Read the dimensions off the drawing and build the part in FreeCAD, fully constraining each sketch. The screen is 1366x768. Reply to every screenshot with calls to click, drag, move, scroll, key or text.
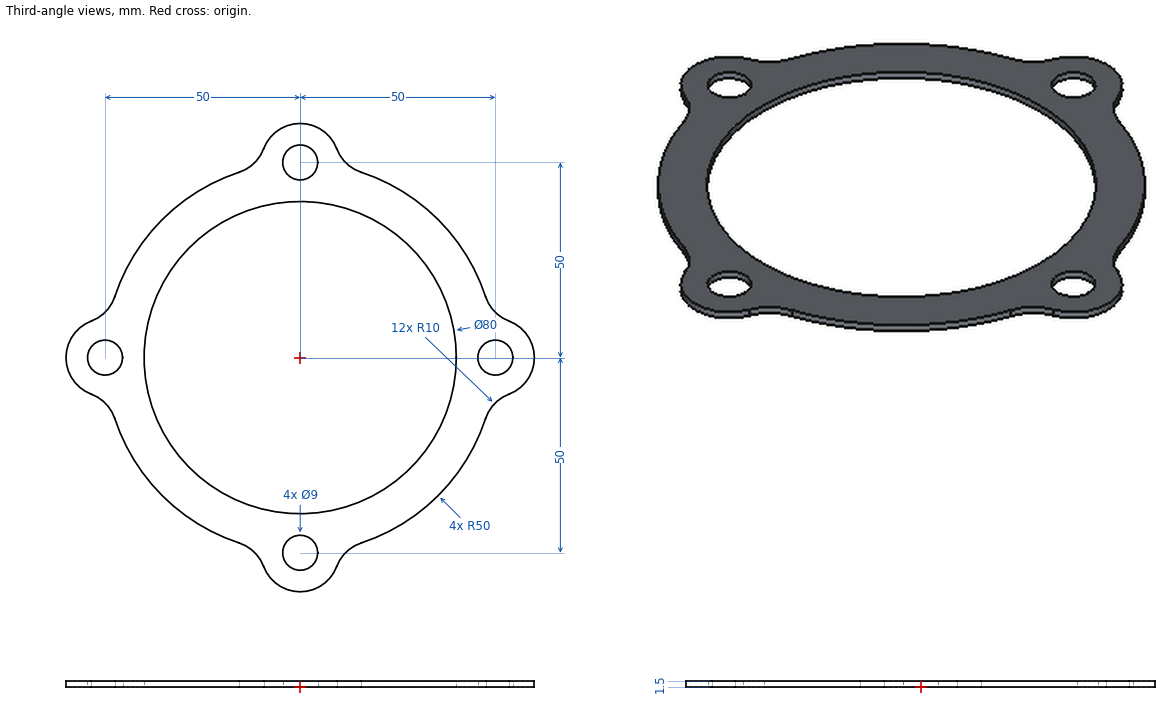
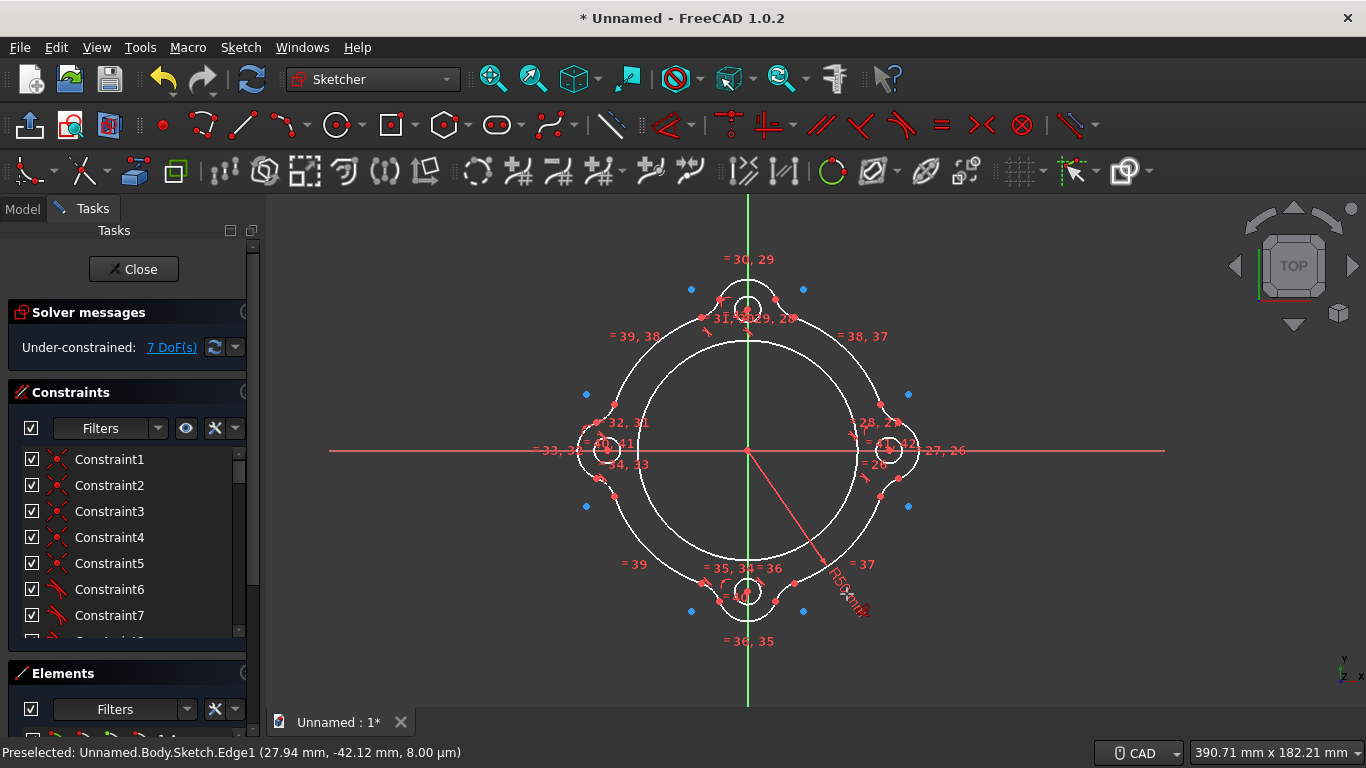
scroll(888, 486, up, 2)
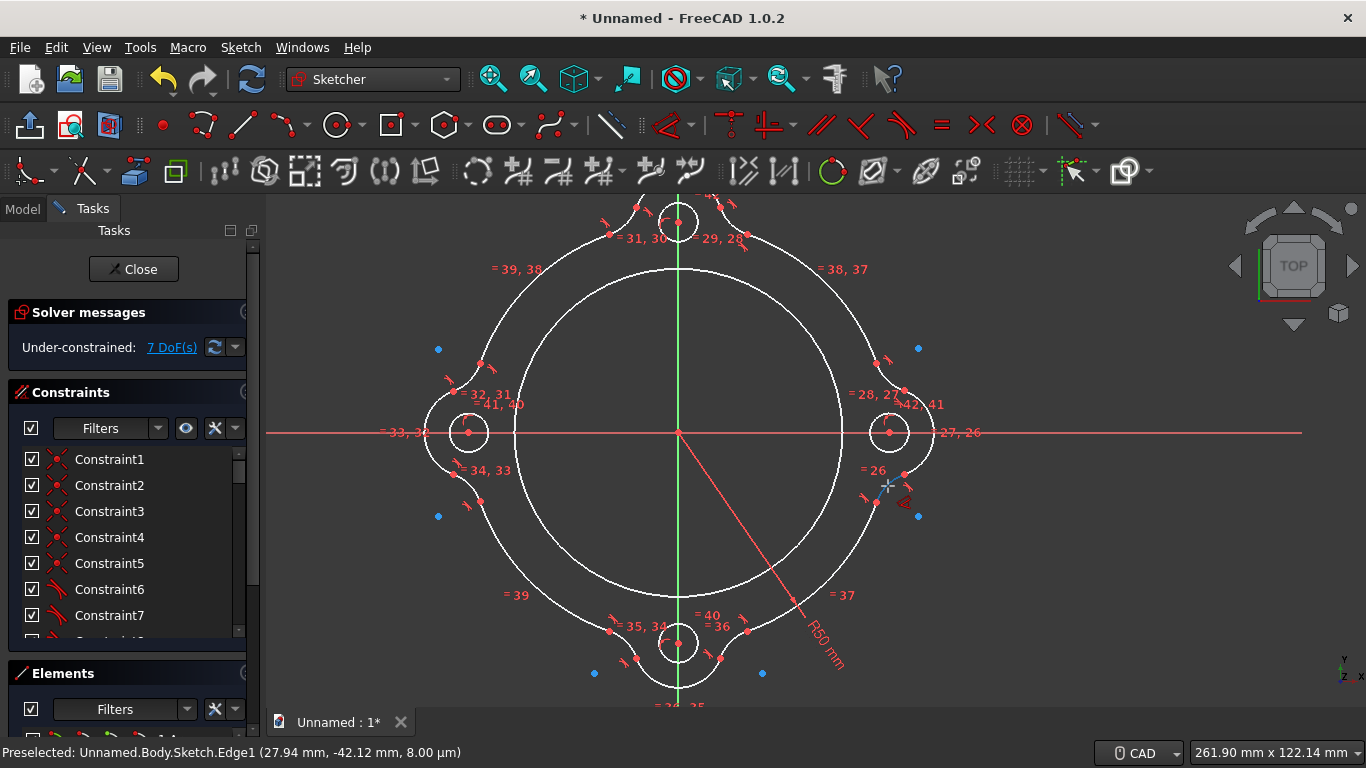
click(887, 485)
click(864, 462)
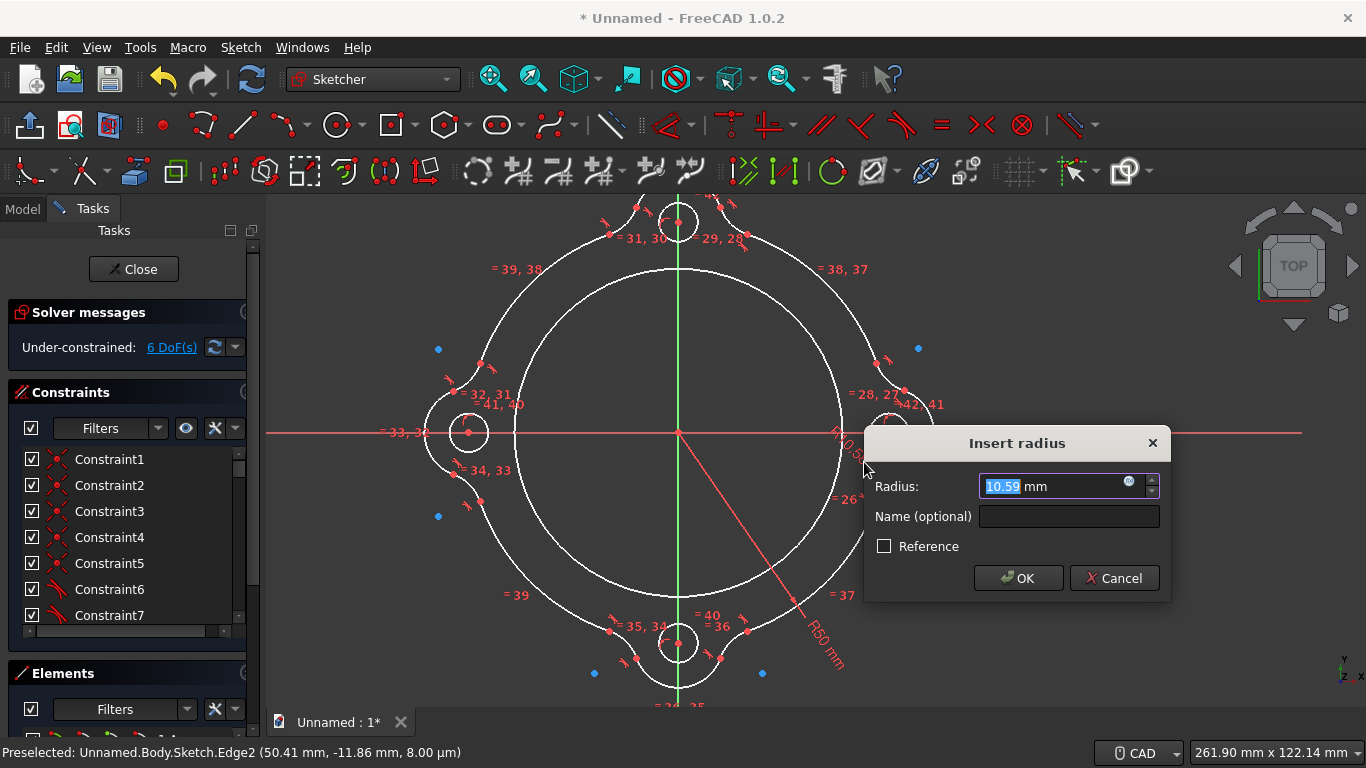
text(10)
key(Return)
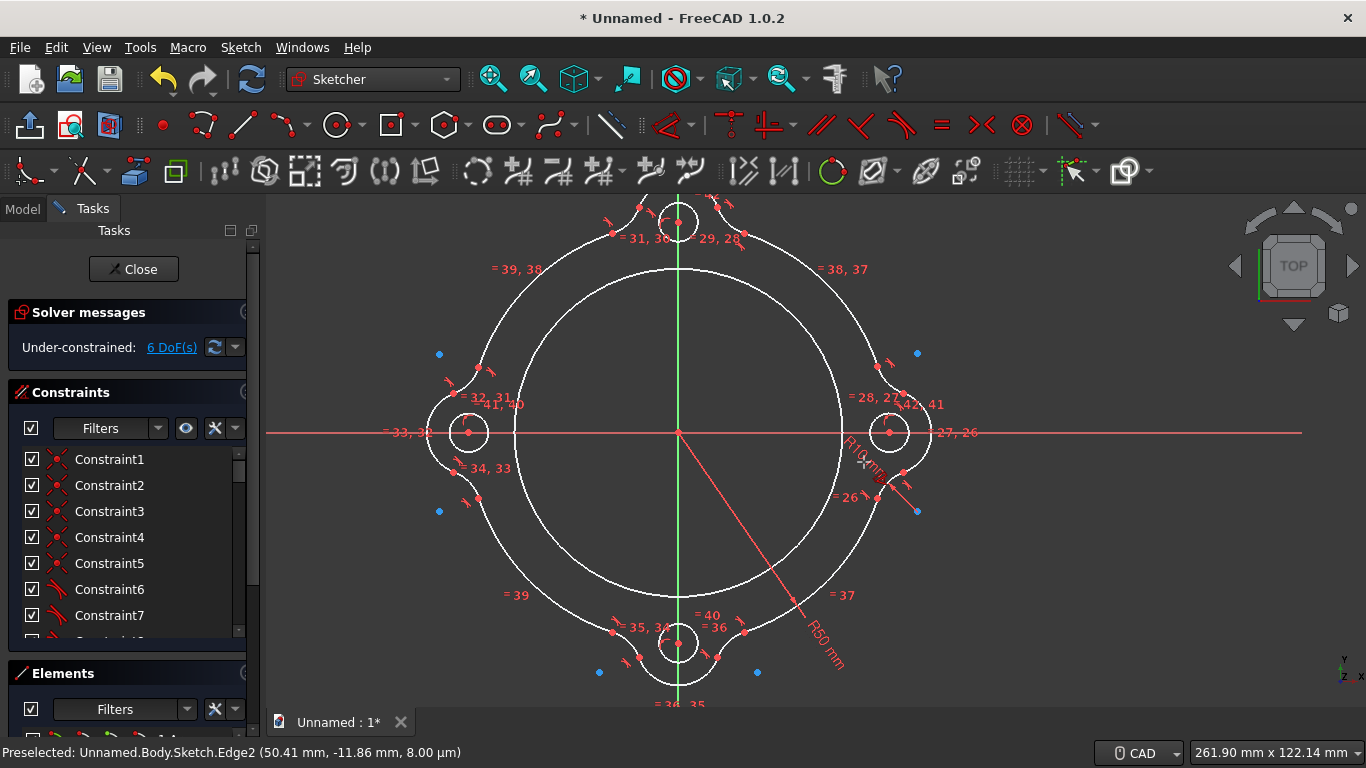
click(692, 630)
click(715, 608)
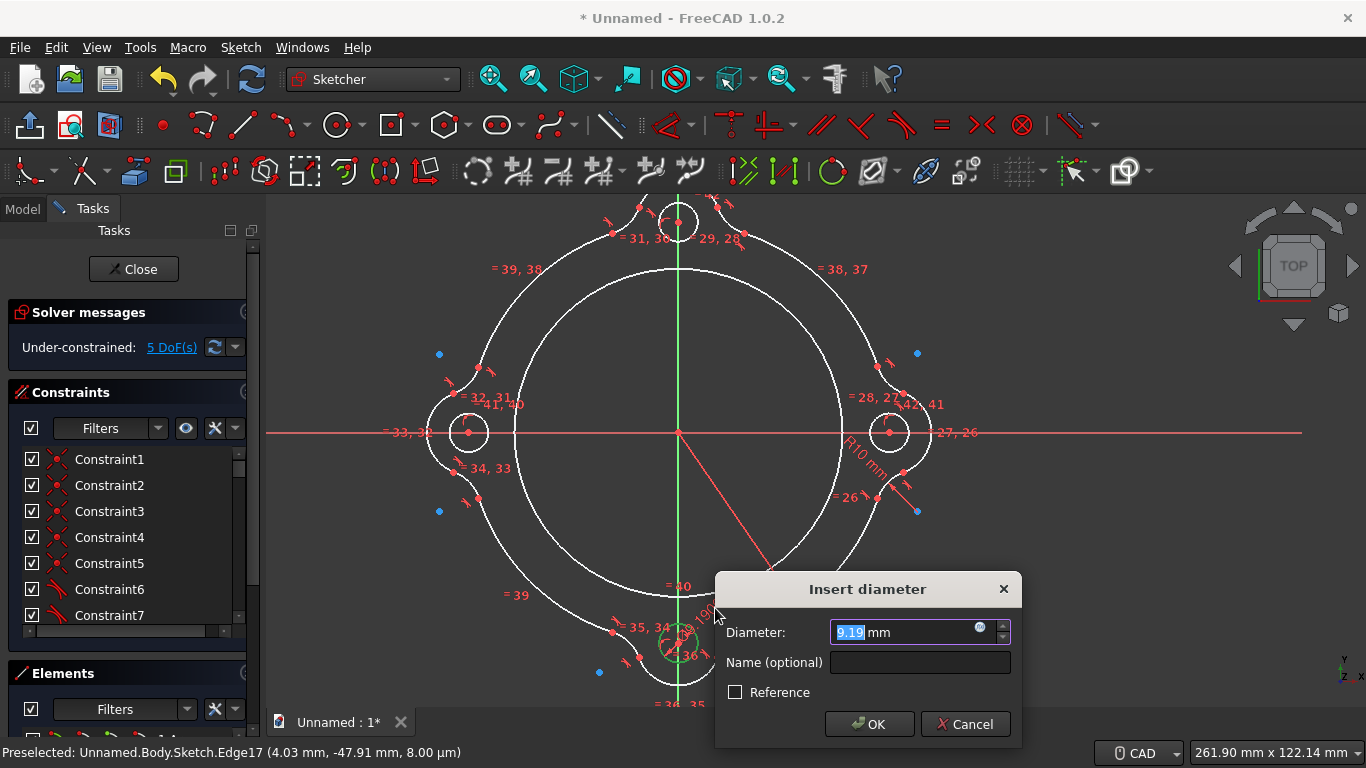
text(9)
key(Return)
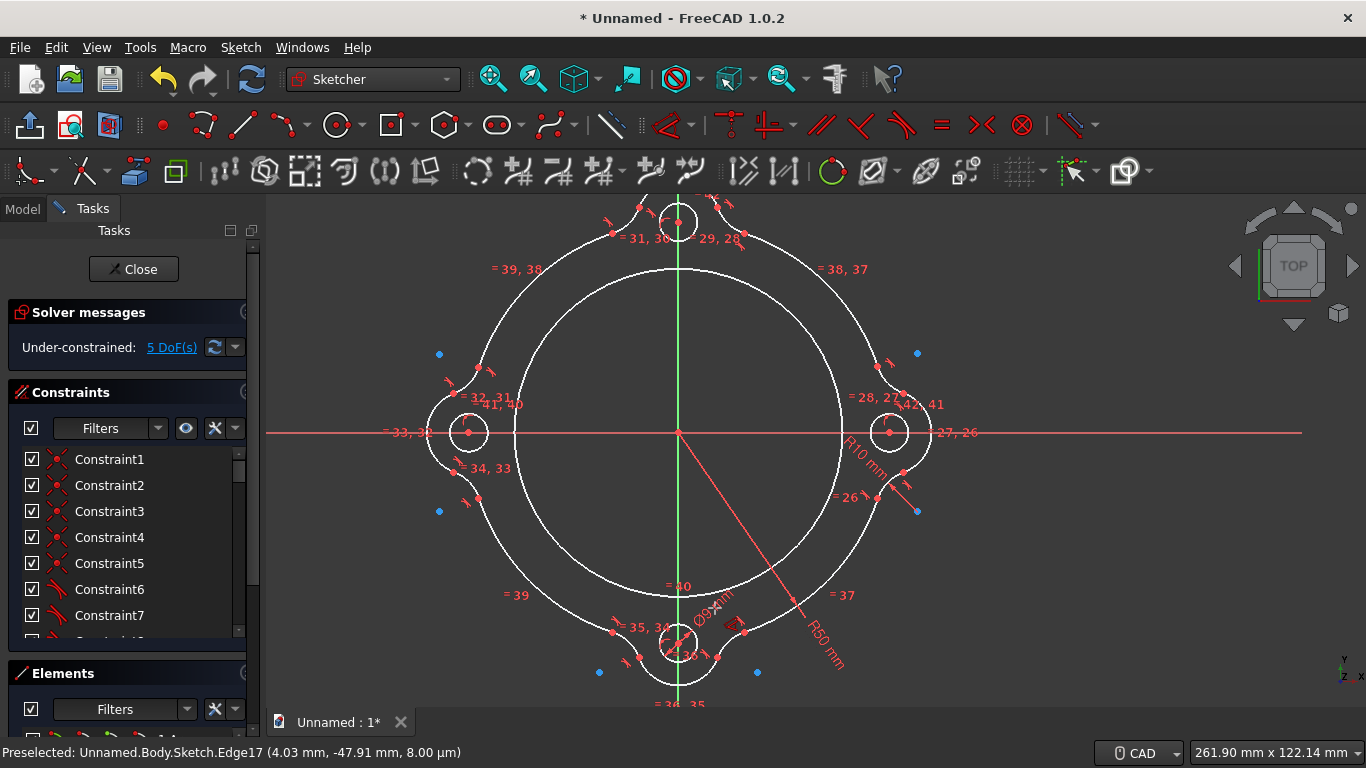
click(794, 316)
click(817, 293)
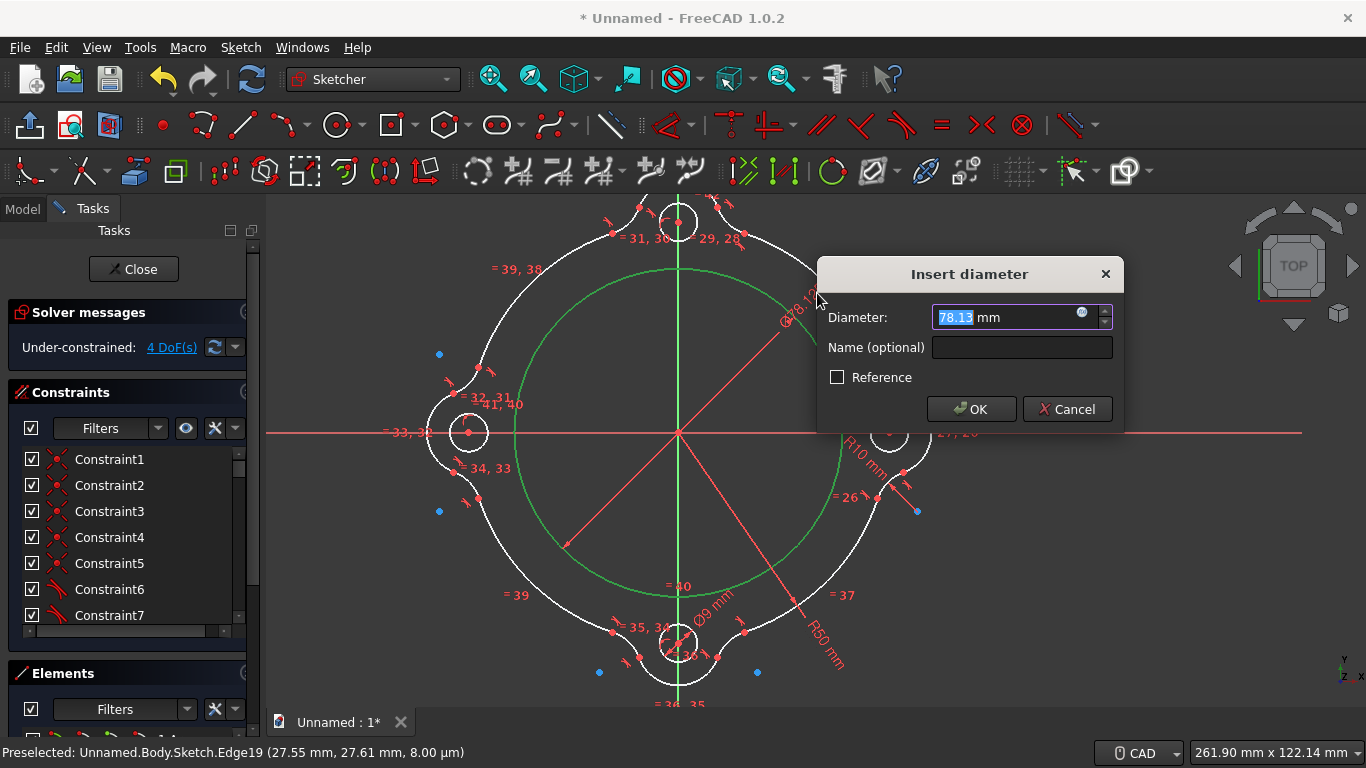
text(80)
key(Return)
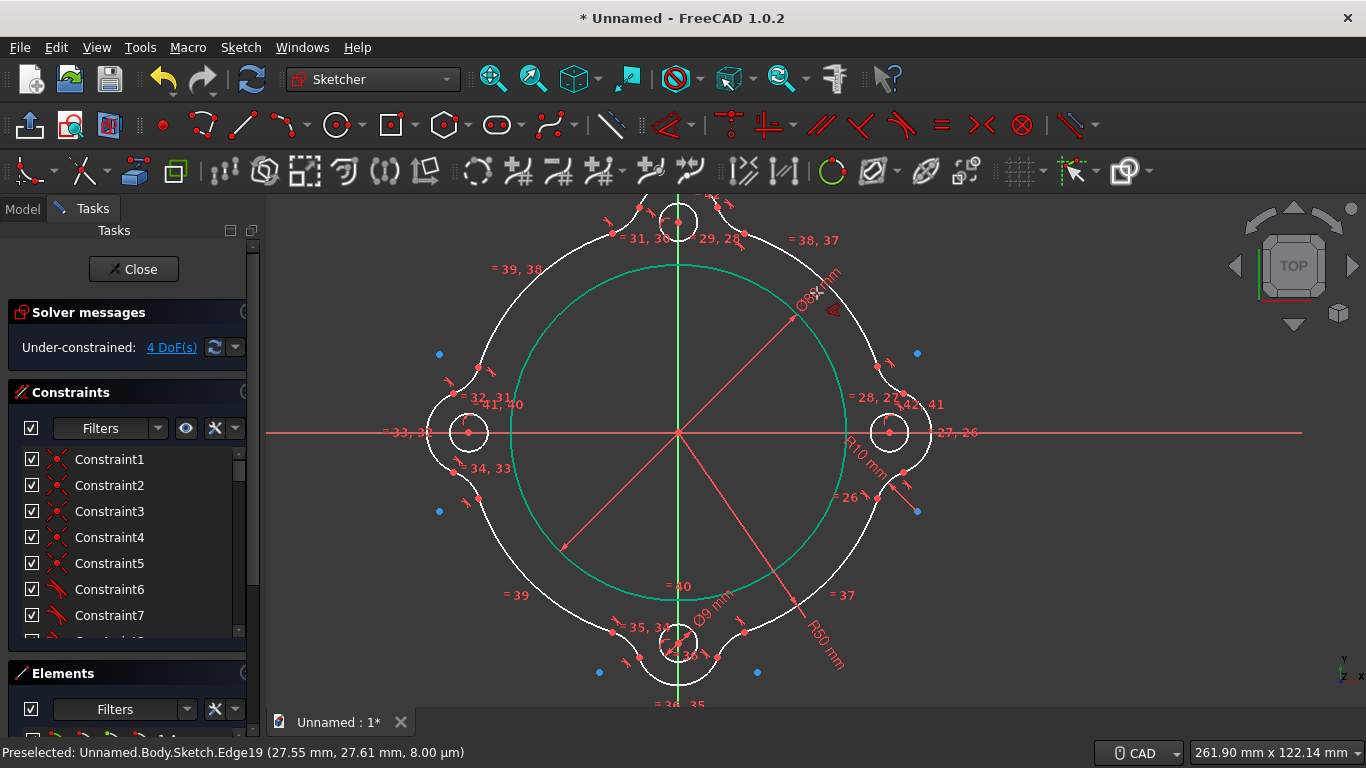
click(678, 643)
click(712, 538)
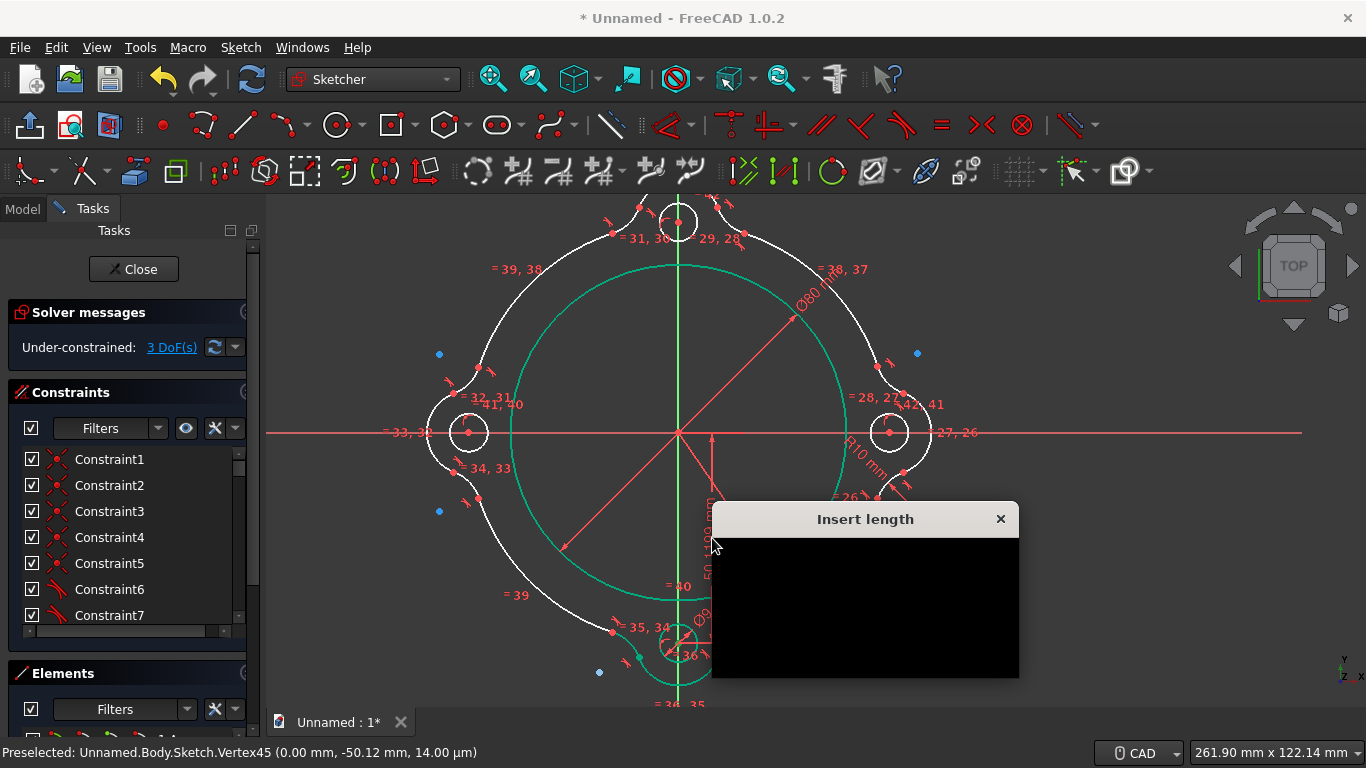
text(50)
key(Return)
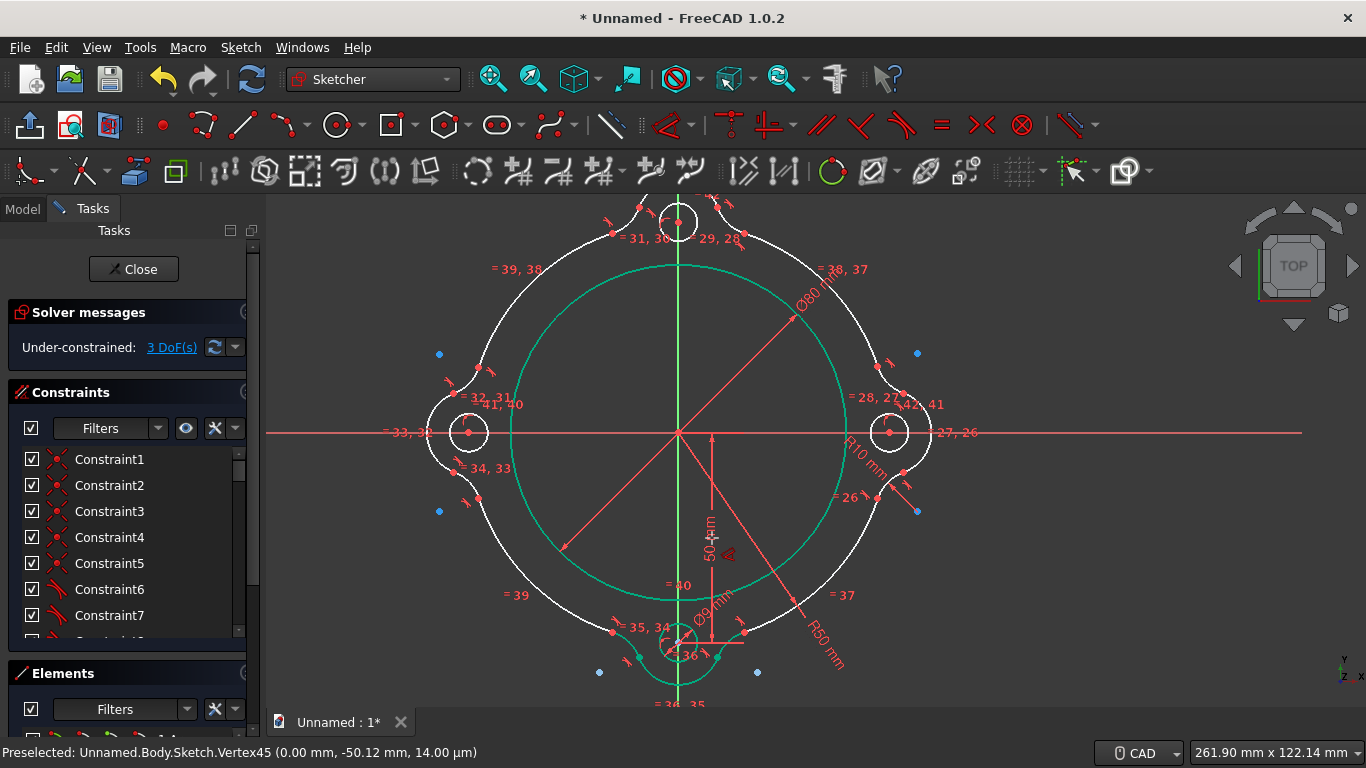
click(469, 433)
click(574, 467)